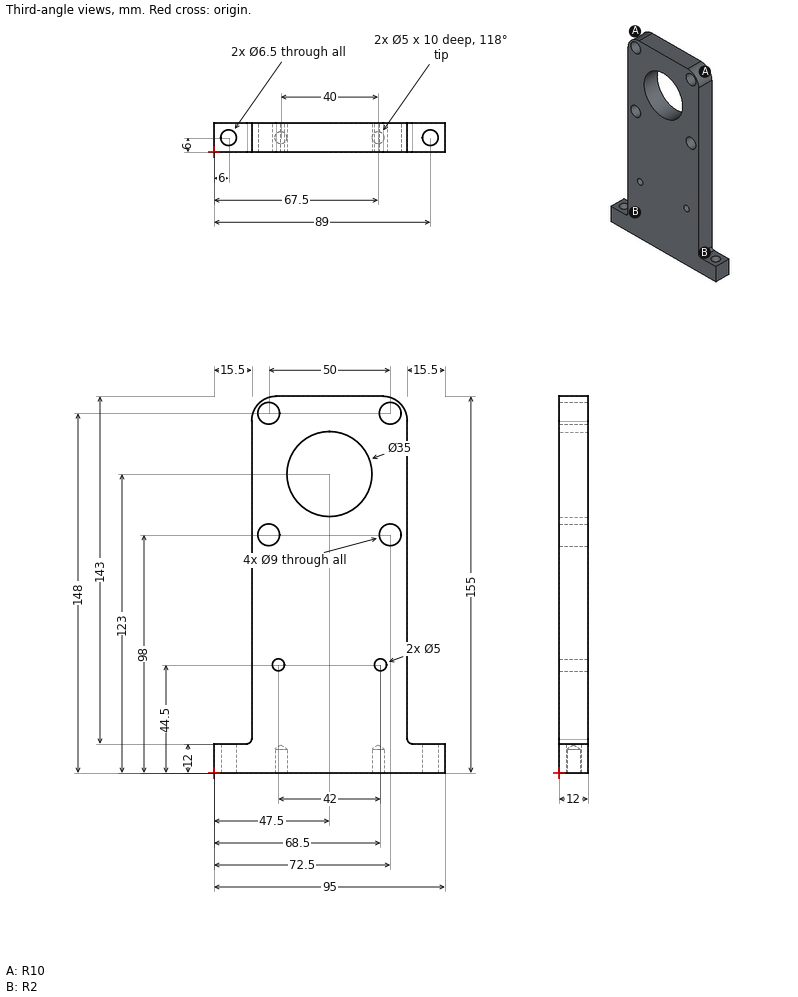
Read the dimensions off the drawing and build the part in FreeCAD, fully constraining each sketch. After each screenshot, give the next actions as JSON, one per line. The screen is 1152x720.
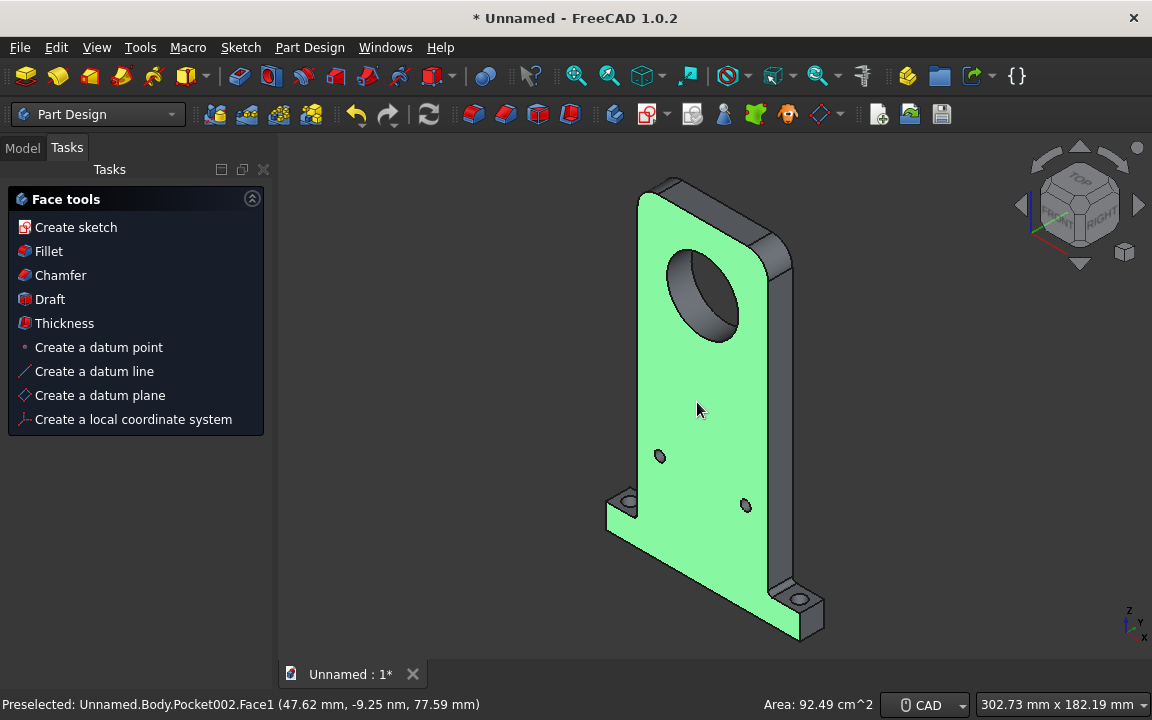
{"action": "left_click", "coordinate": [648, 114]}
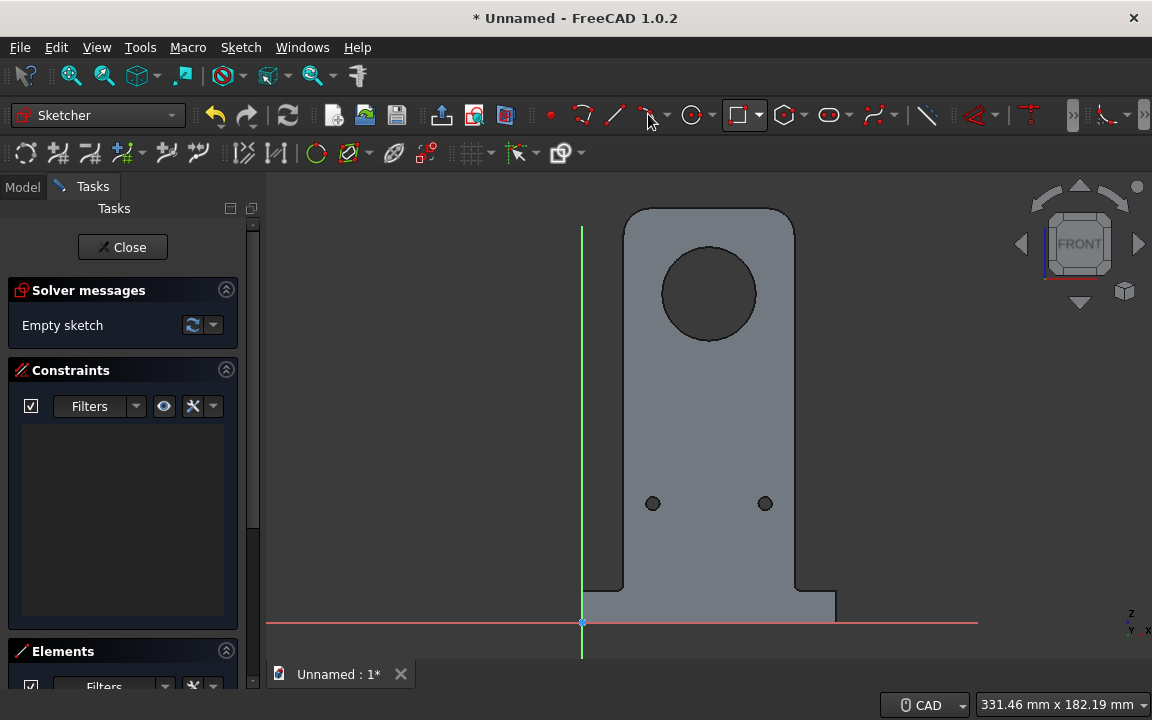
{"action": "scroll", "coordinate": [792, 200], "scroll_direction": "up", "scroll_amount": 3}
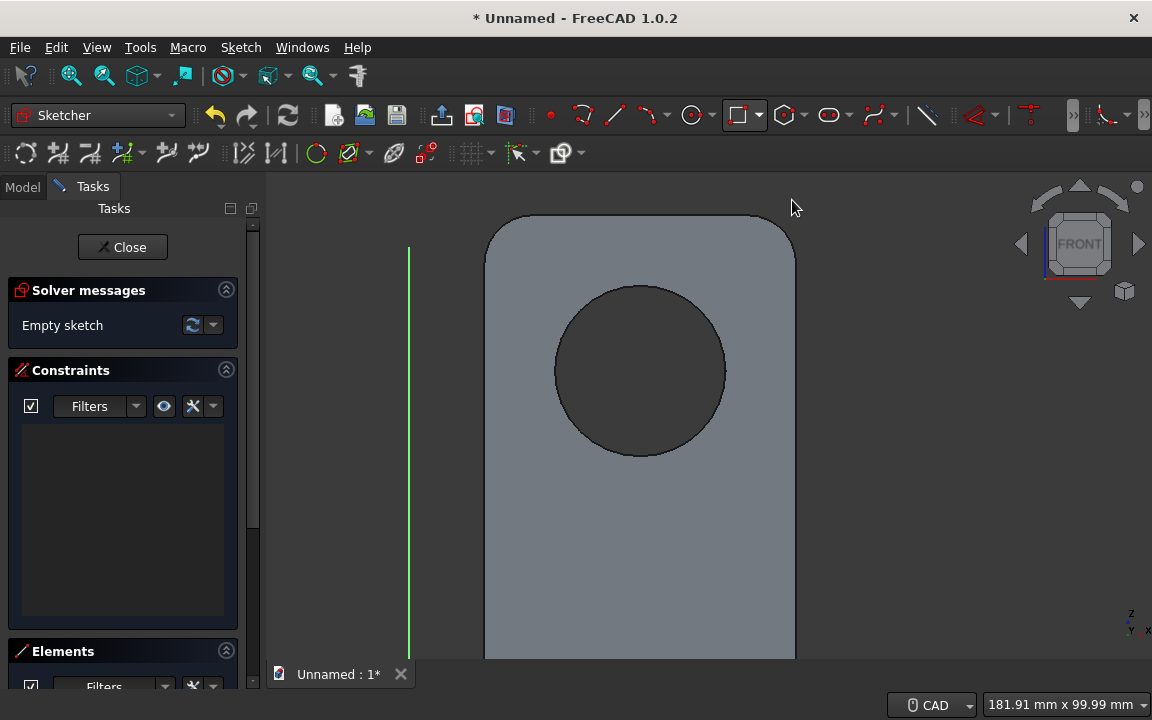
{"action": "left_click", "coordinate": [692, 116]}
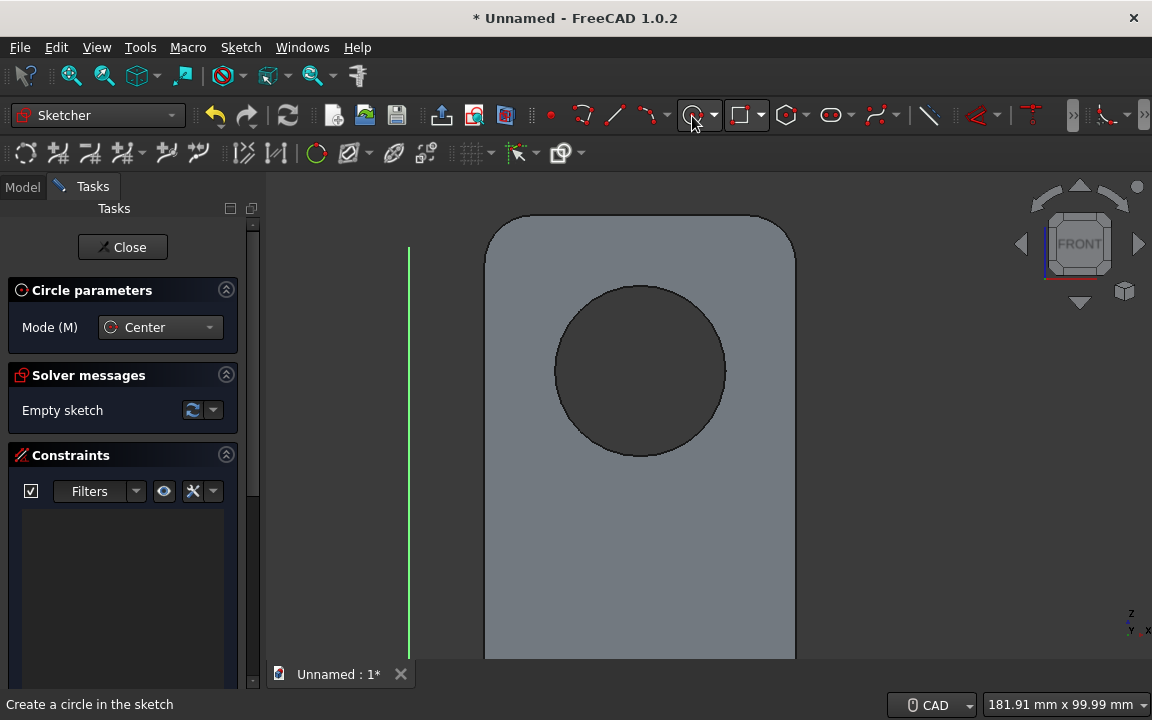
{"action": "left_click", "coordinate": [762, 493]}
{"action": "left_click", "coordinate": [778, 477]}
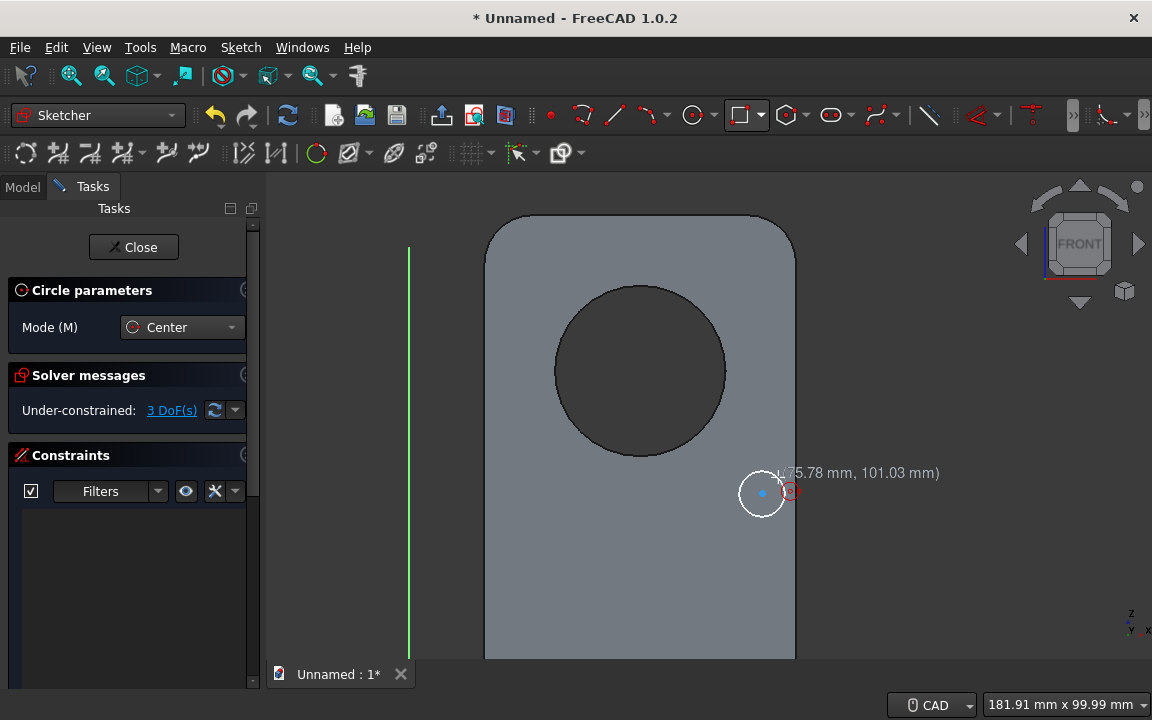
{"action": "left_click", "coordinate": [762, 249]}
{"action": "left_click", "coordinate": [778, 234]}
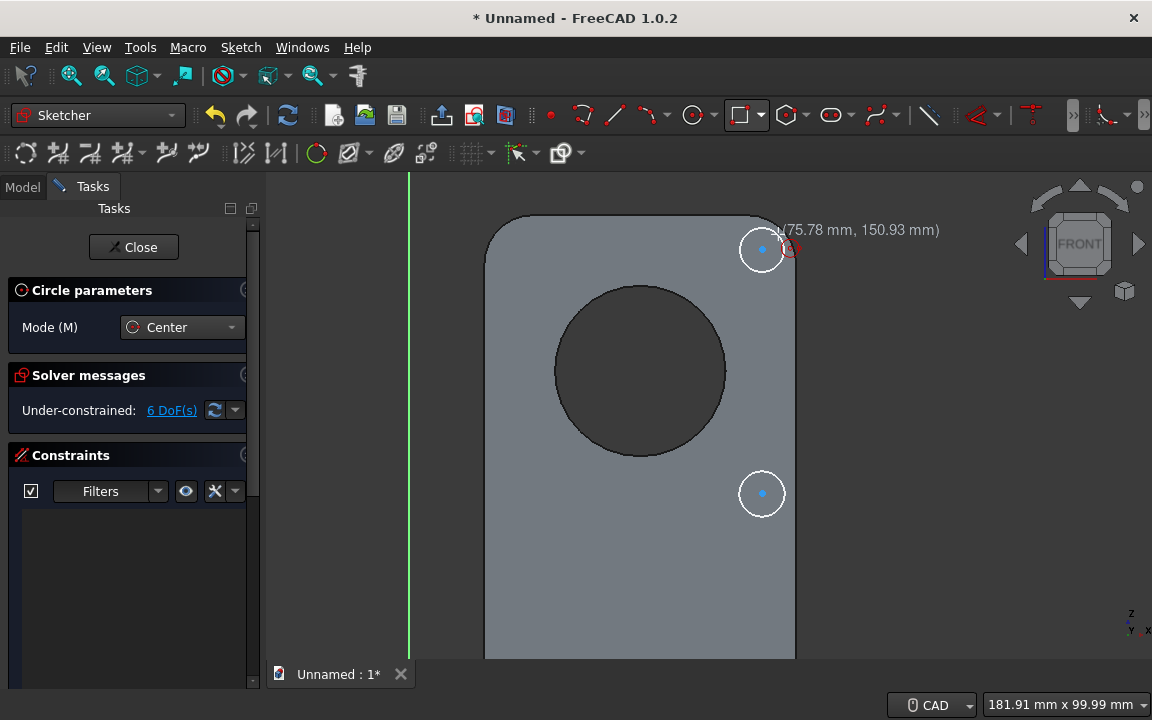
{"action": "left_click", "coordinate": [519, 249]}
{"action": "left_click", "coordinate": [534, 234]}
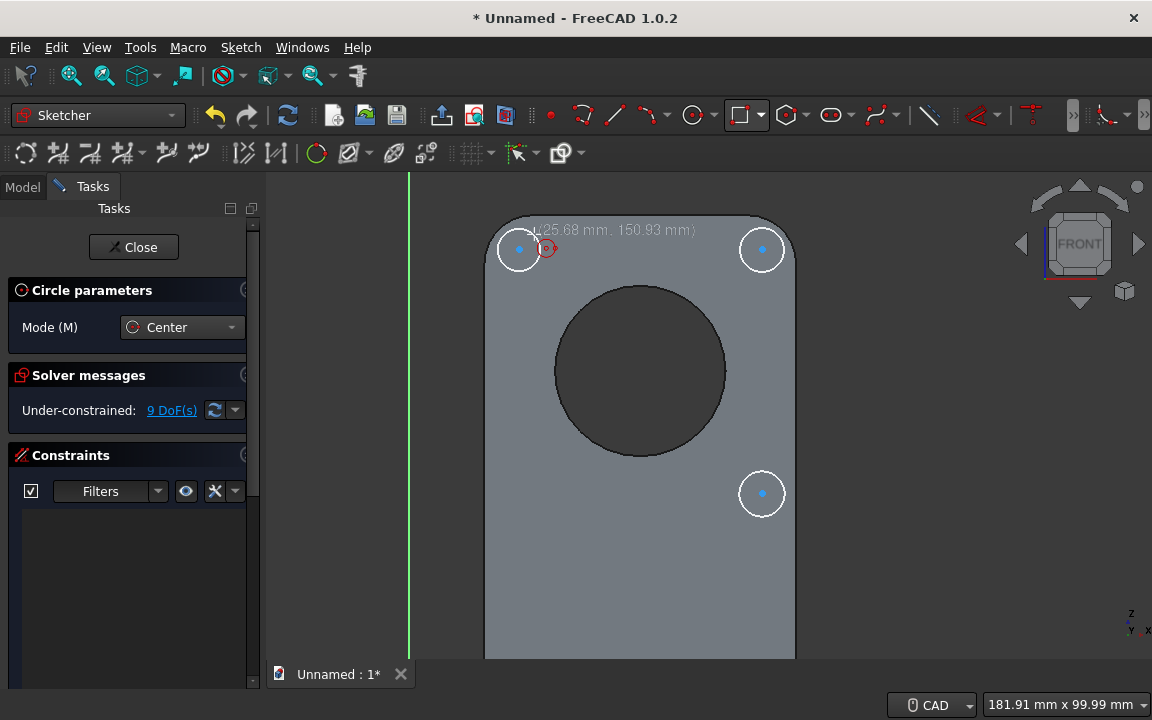
{"action": "left_click", "coordinate": [519, 493]}
{"action": "left_click", "coordinate": [534, 477]}
{"action": "key", "text": "Escape"}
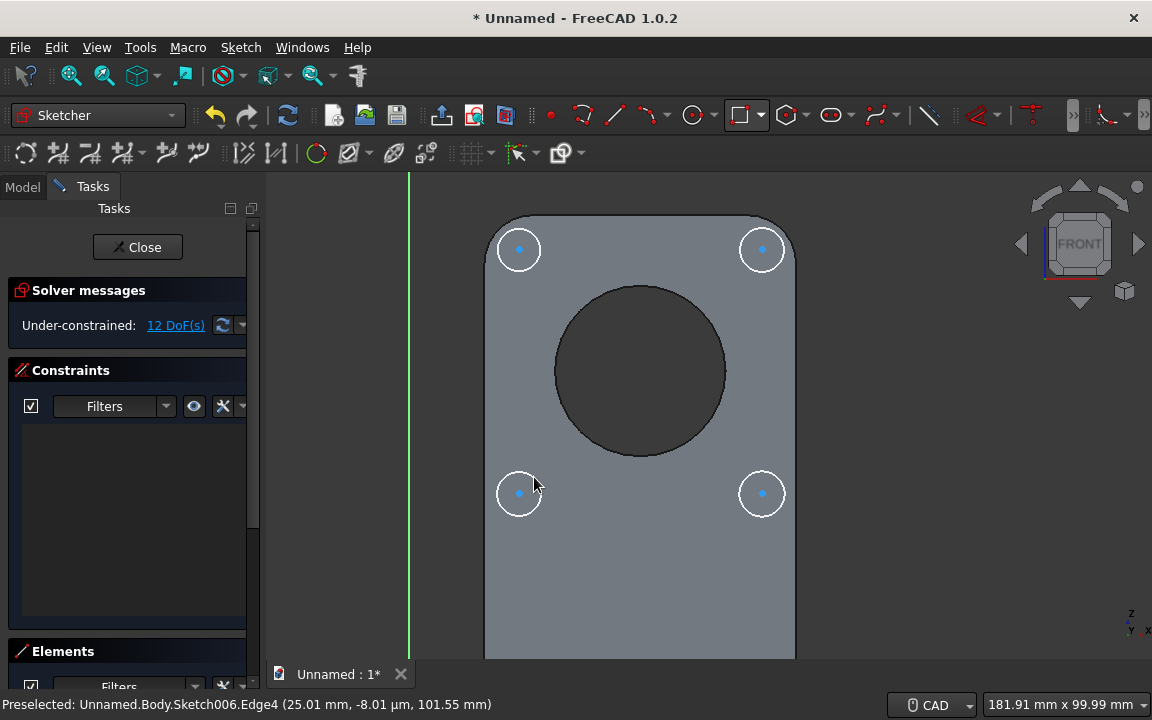
{"action": "left_click", "coordinate": [778, 478]}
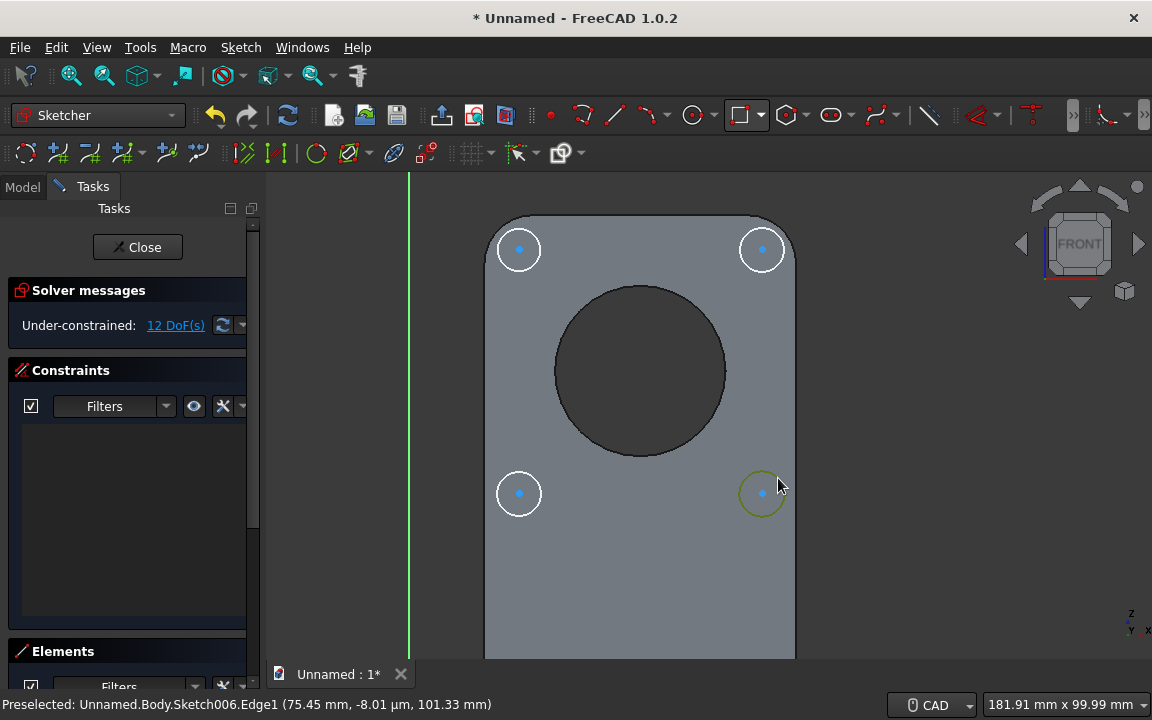
{"action": "left_click", "coordinate": [777, 234]}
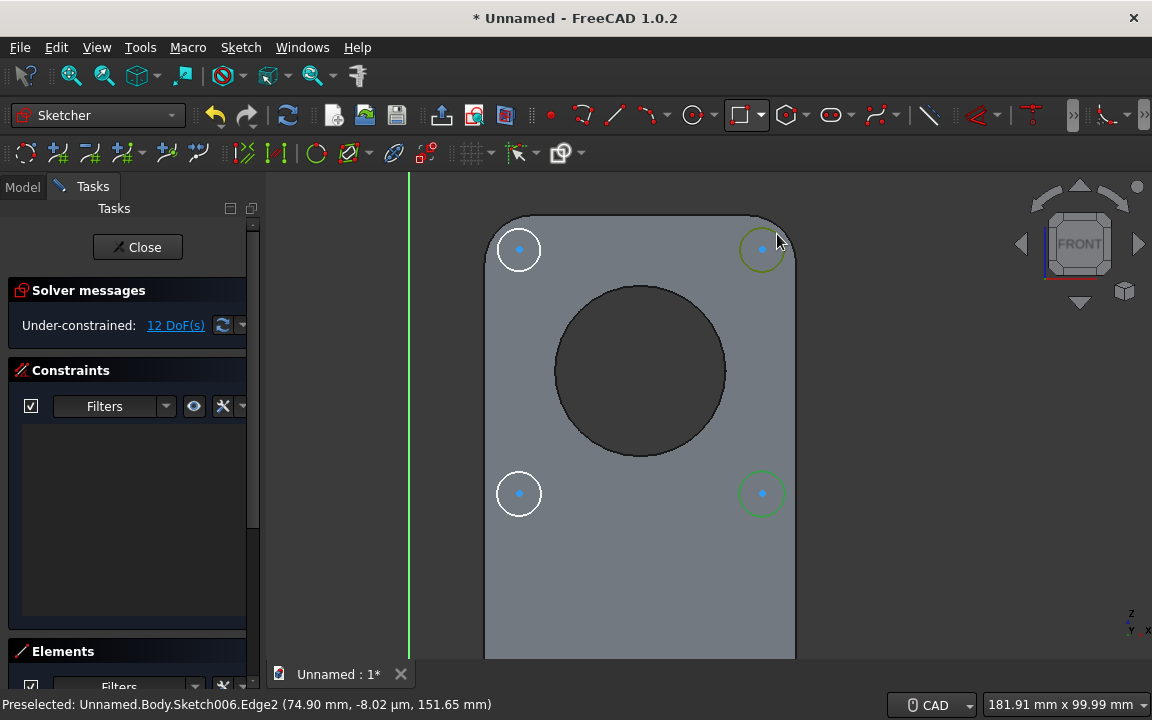
{"action": "left_click", "coordinate": [534, 235]}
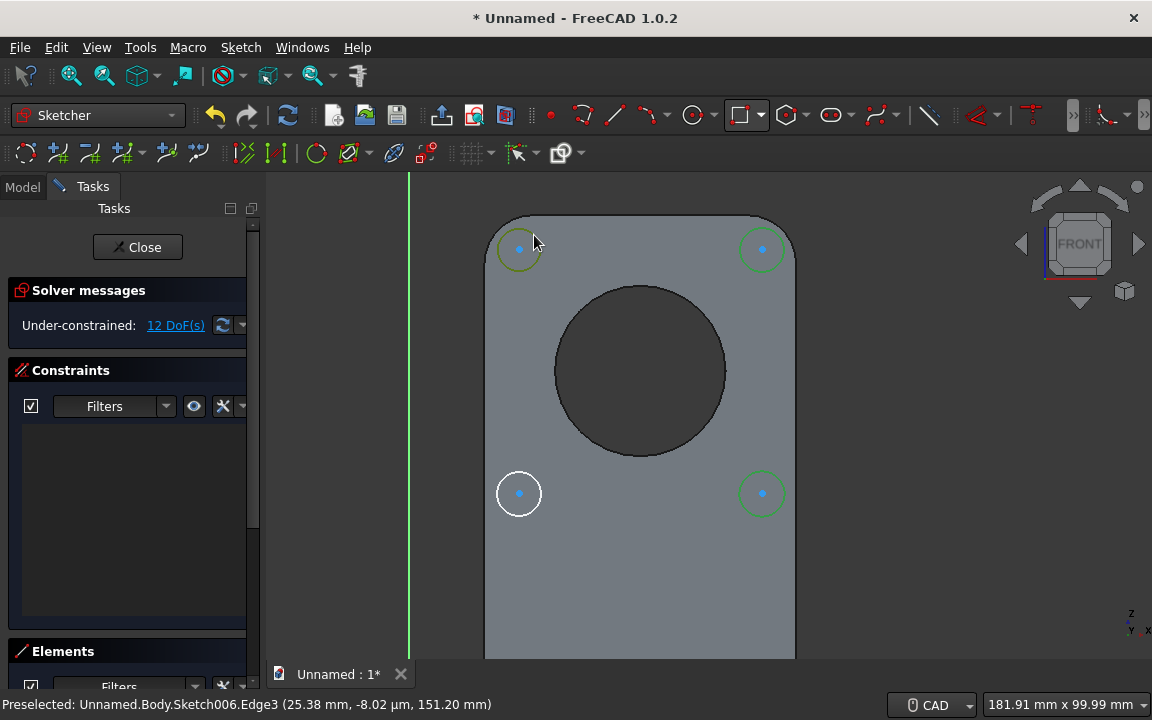
{"action": "left_click", "coordinate": [534, 478]}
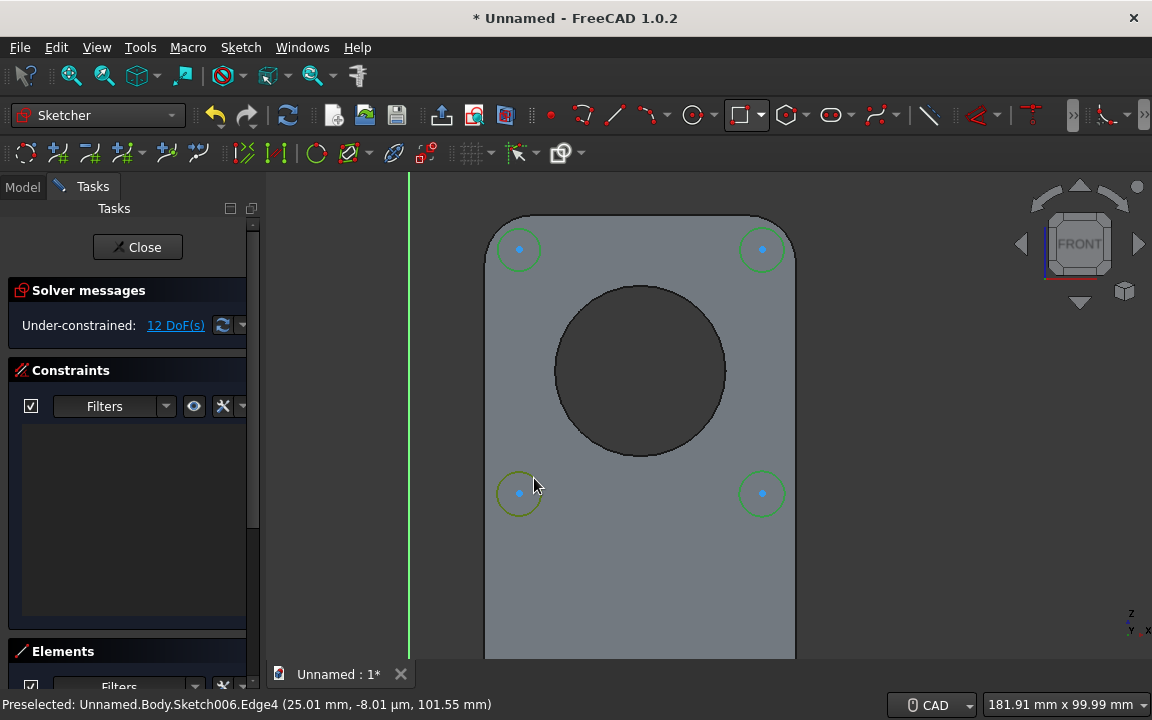
{"action": "key", "text": "e"}